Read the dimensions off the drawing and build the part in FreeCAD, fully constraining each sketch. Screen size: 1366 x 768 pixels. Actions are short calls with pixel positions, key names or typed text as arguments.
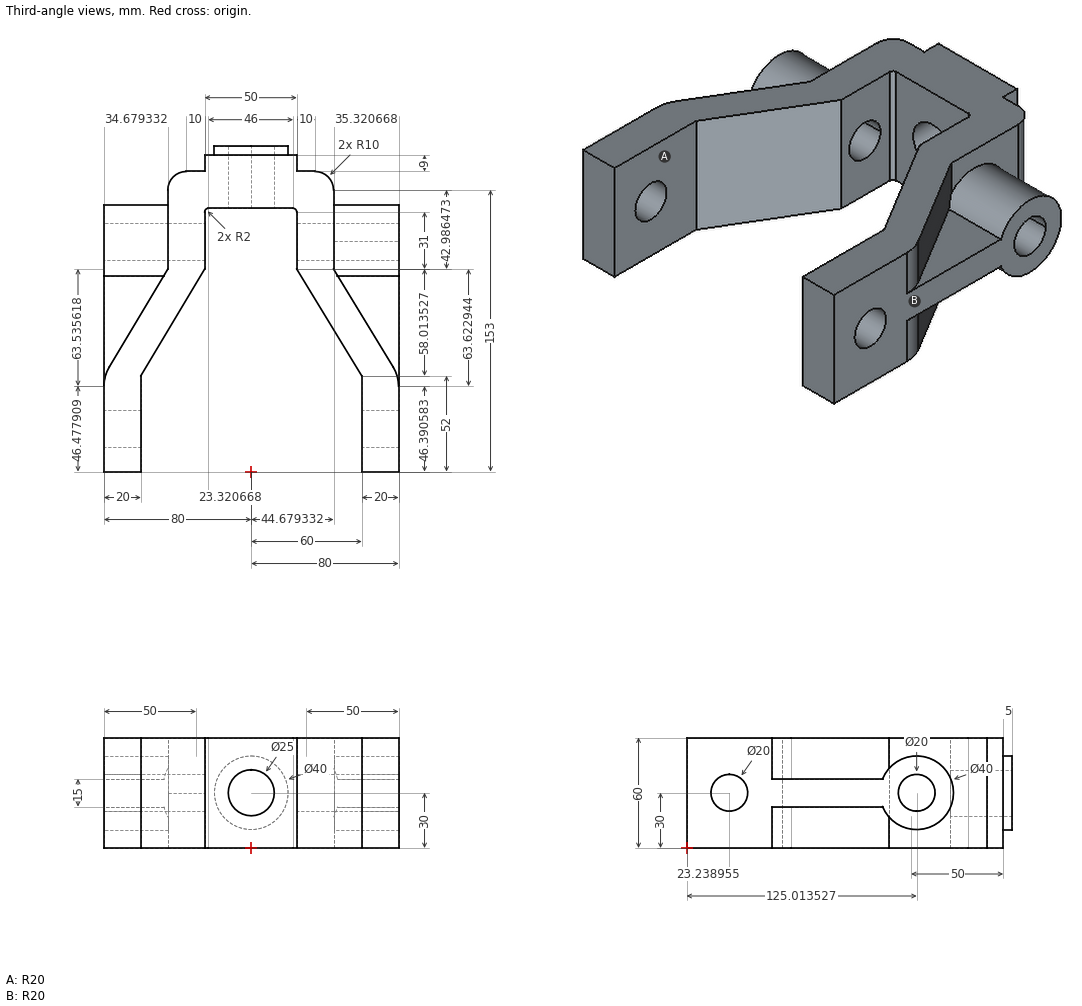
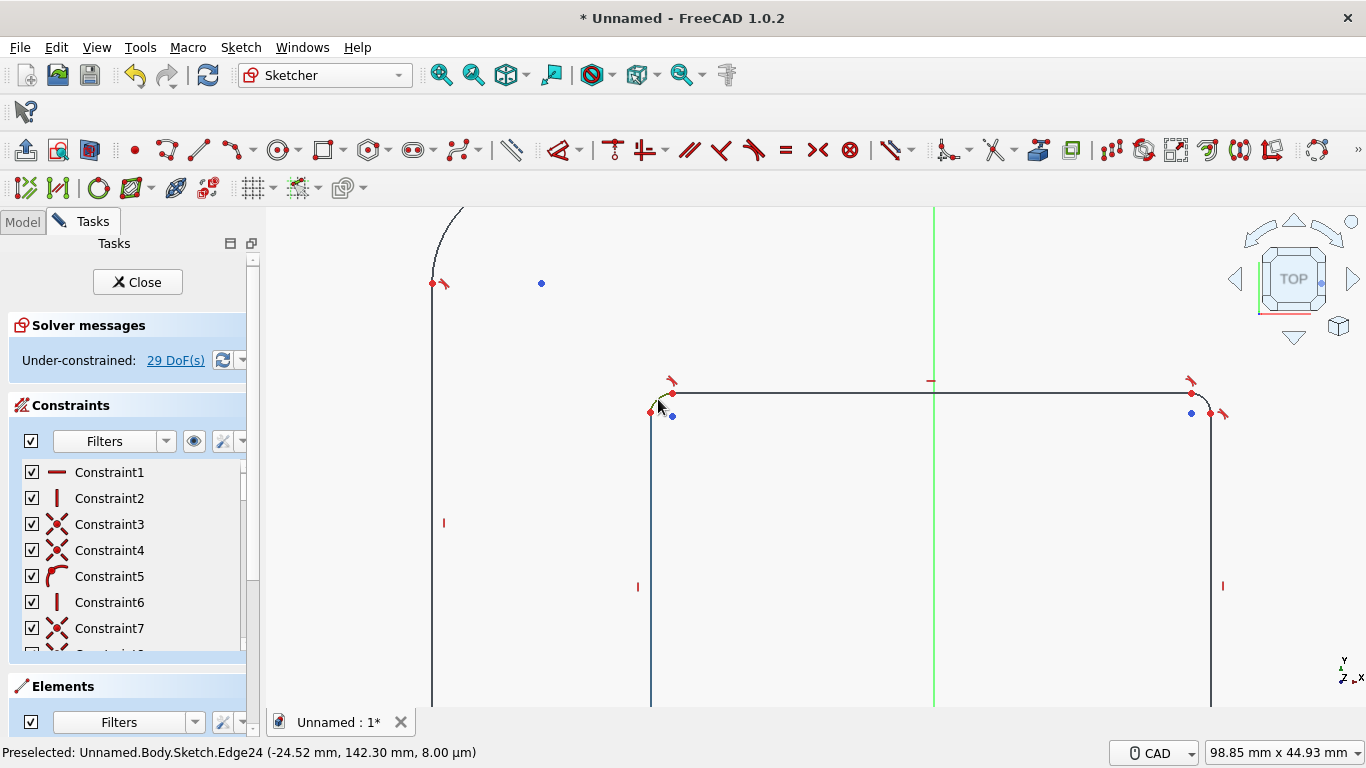
key(t)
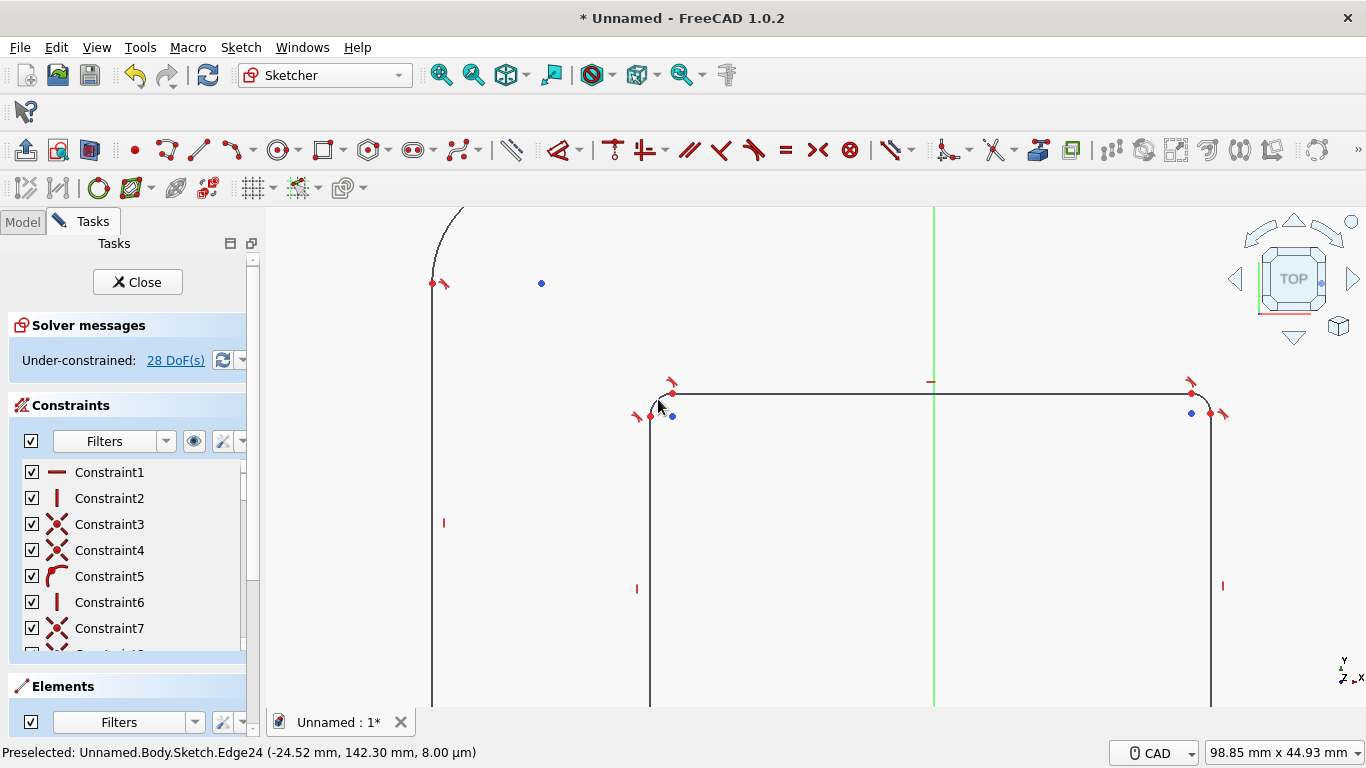
scroll(711, 345, down, 9)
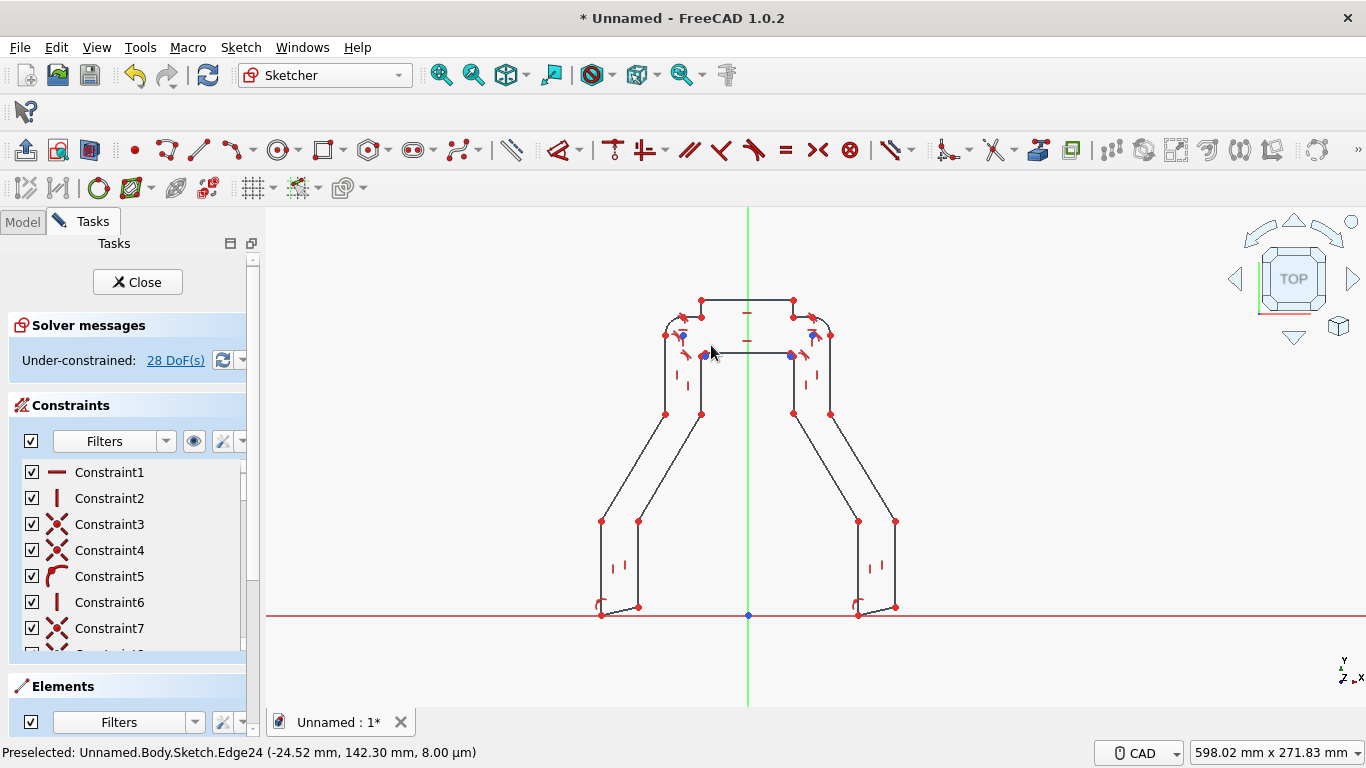
scroll(869, 613, up, 9)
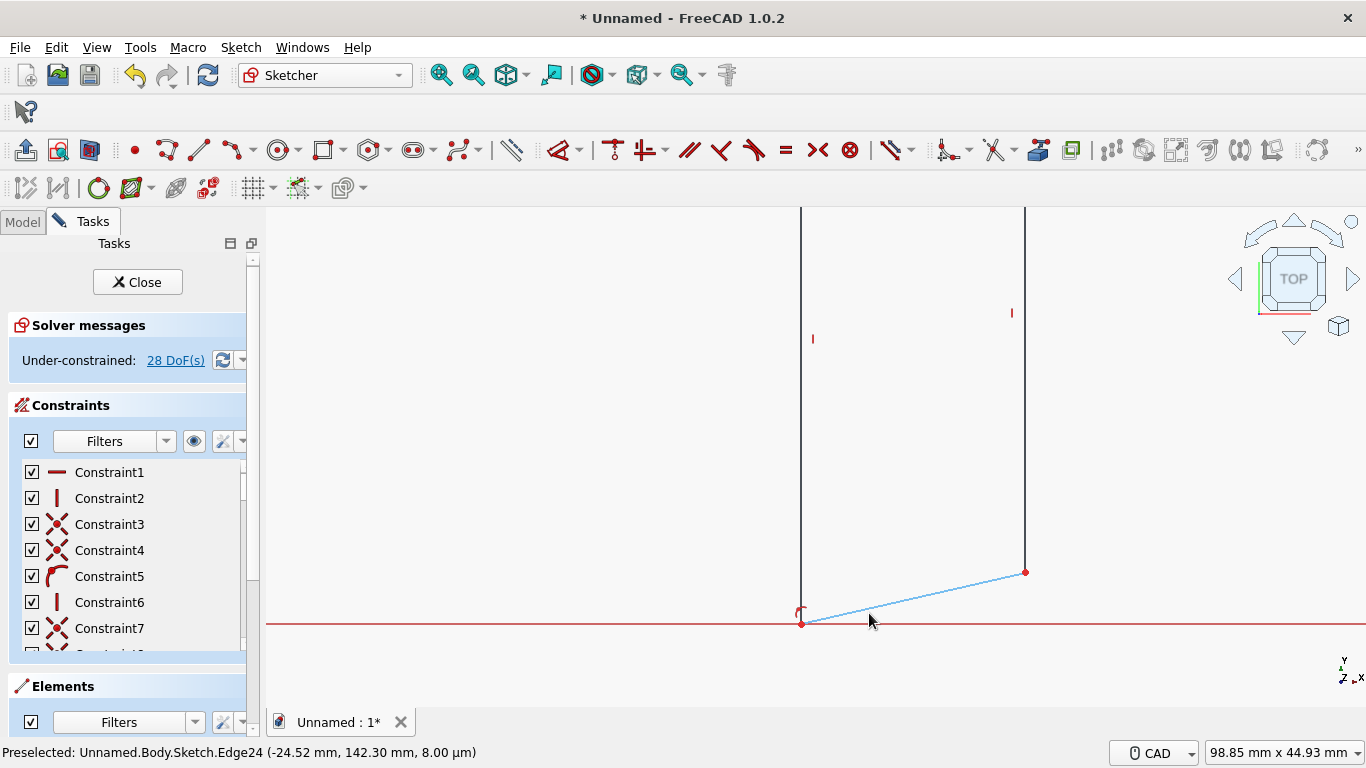
click(868, 609)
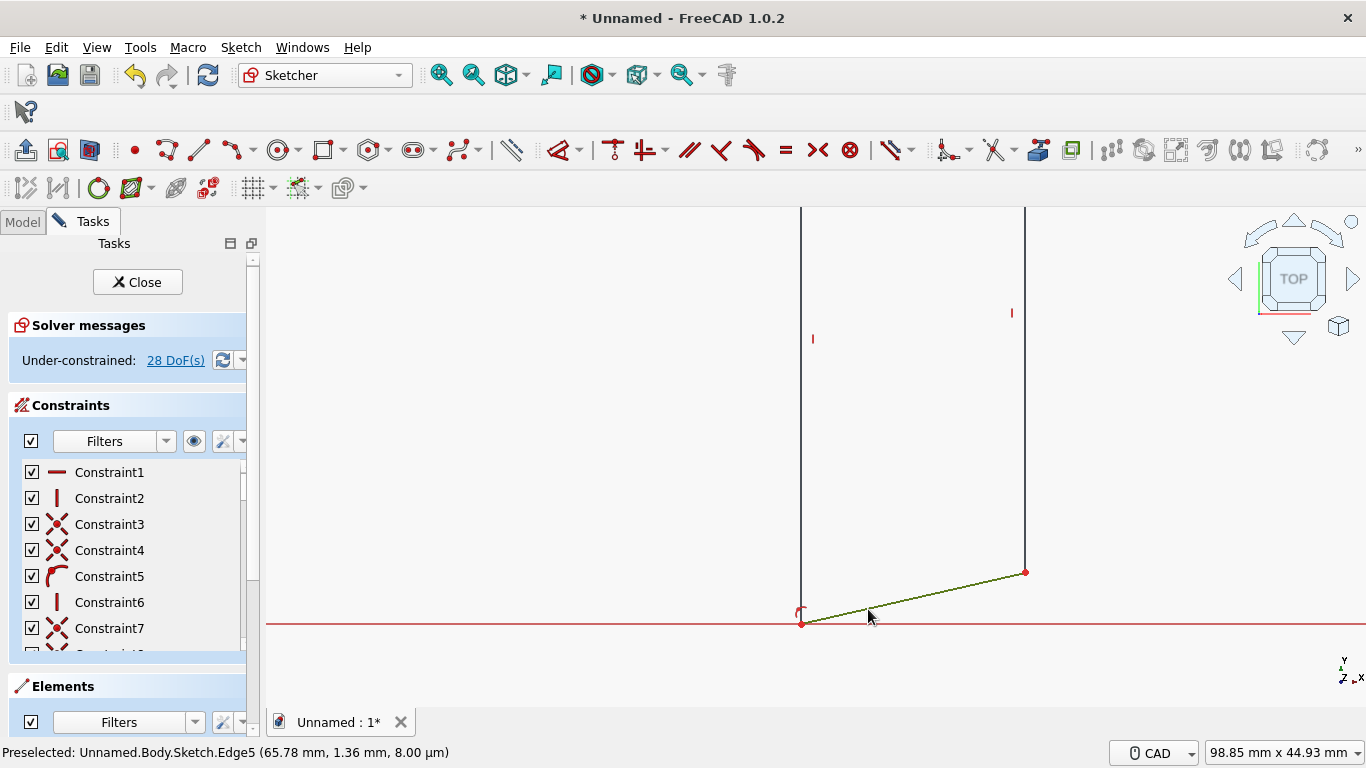
key(h)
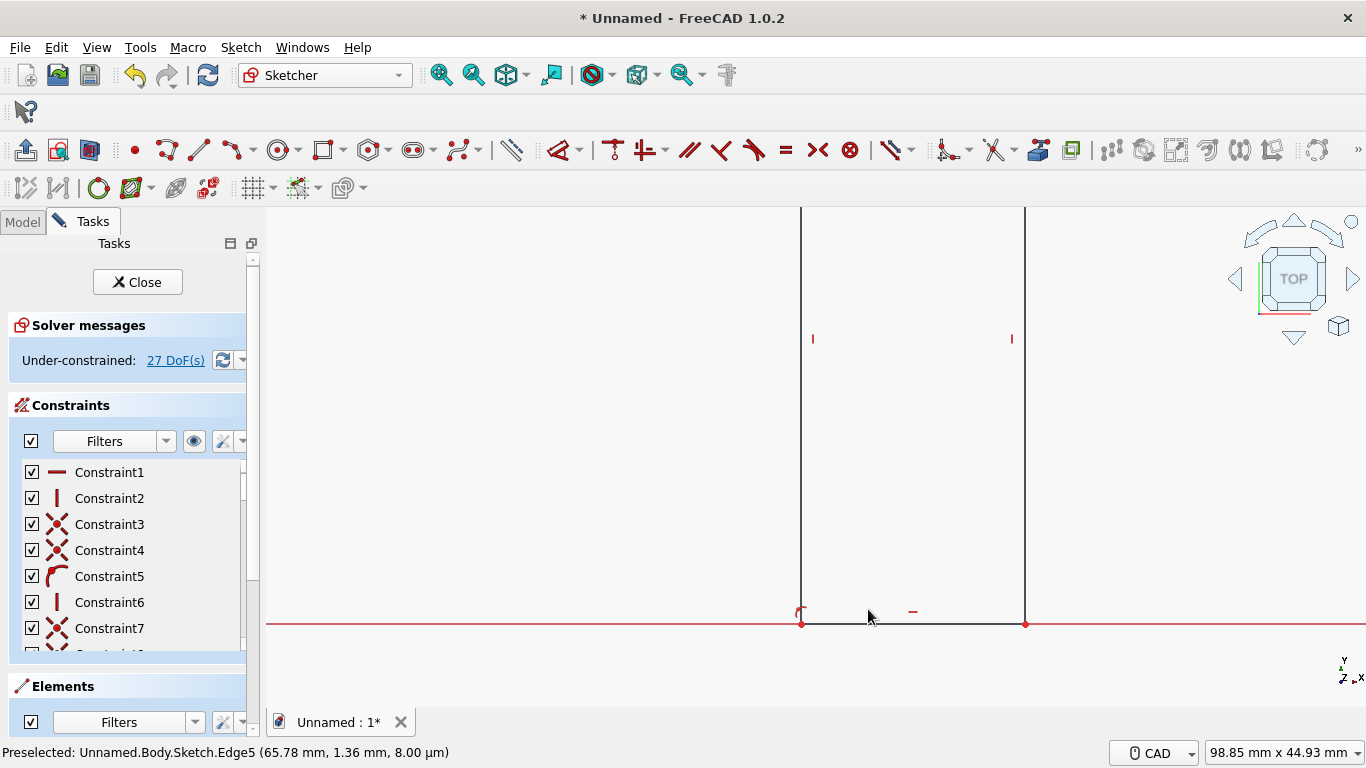
scroll(869, 613, down, 9)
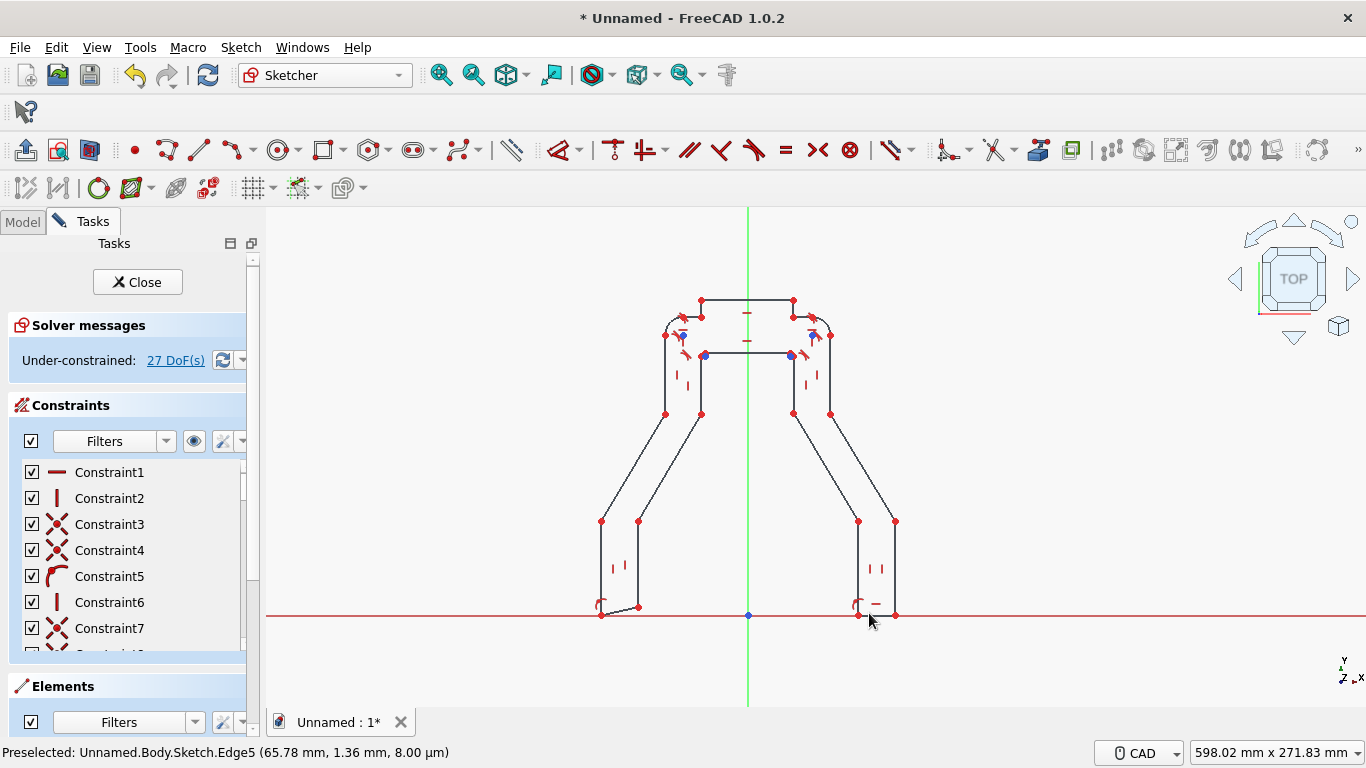
scroll(612, 613, up, 9)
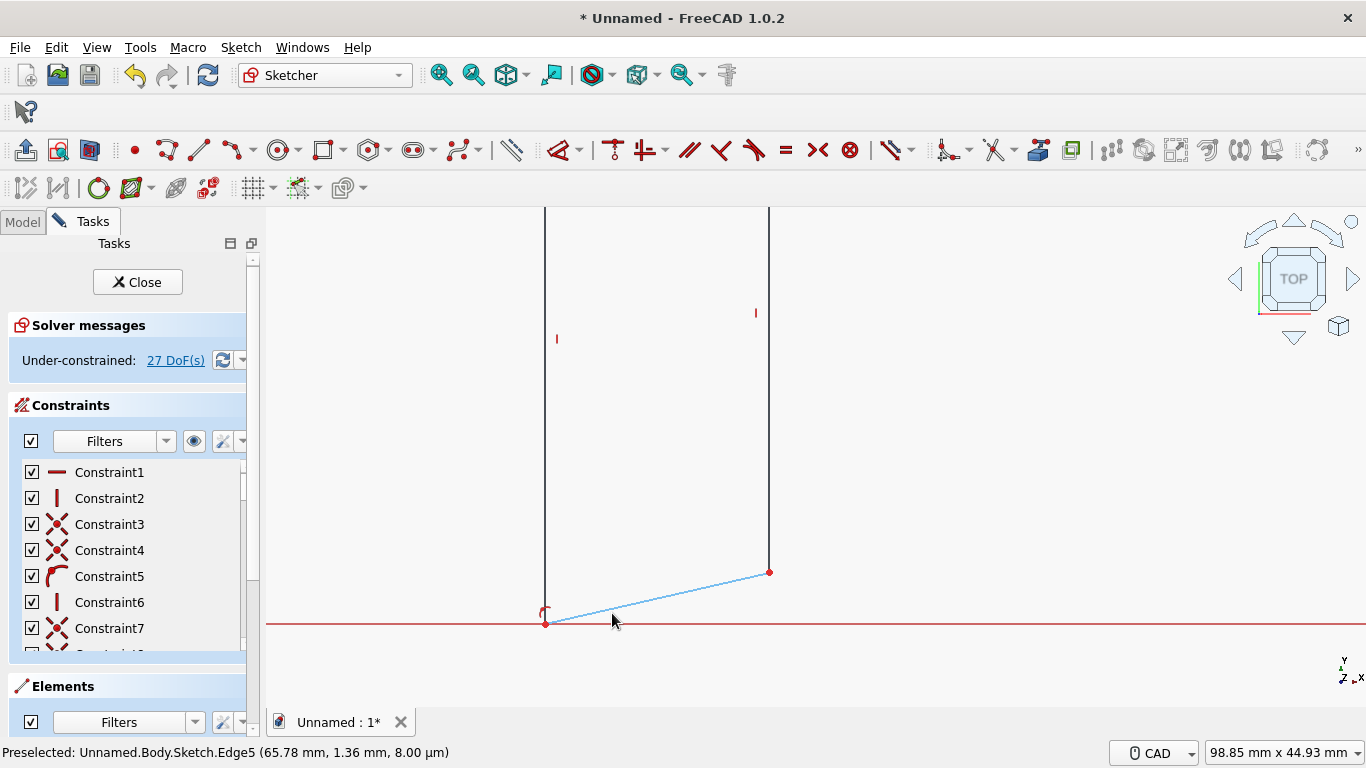
click(613, 609)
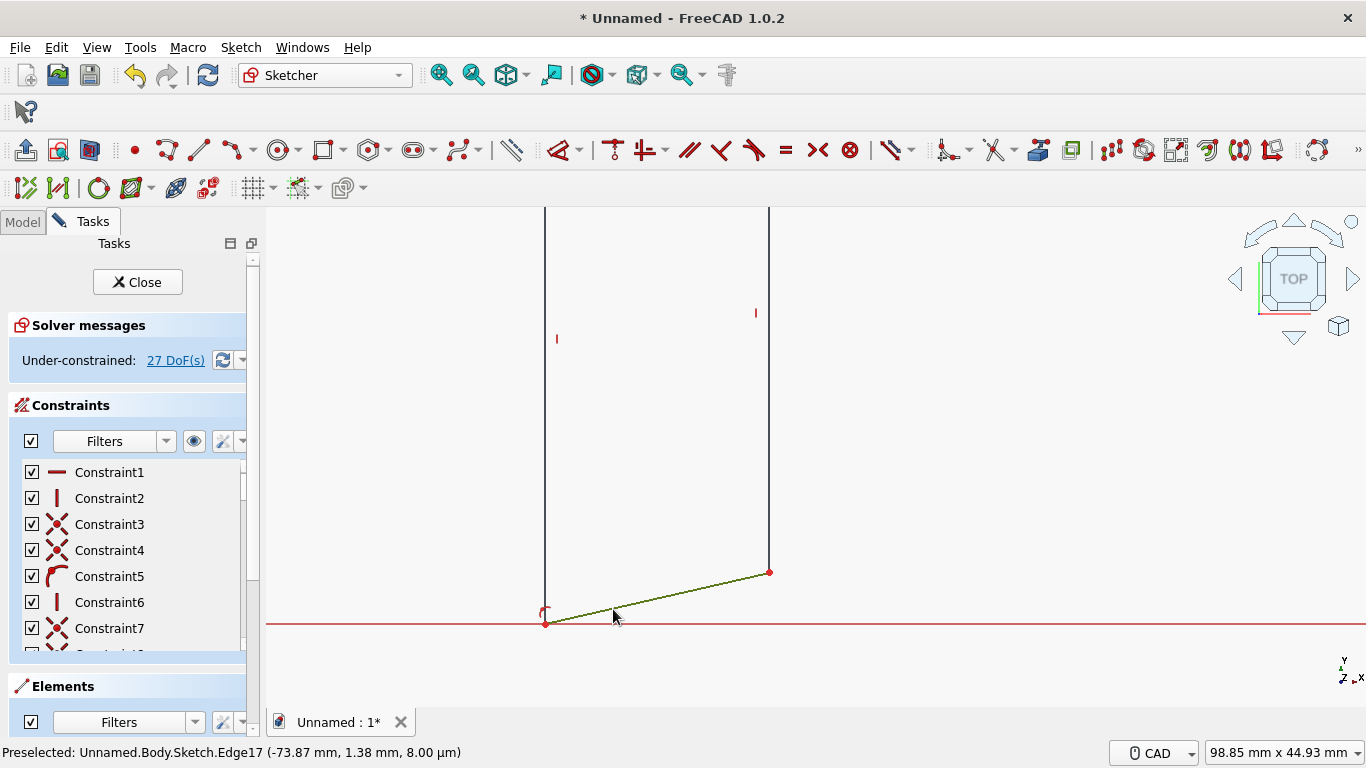
key(h)